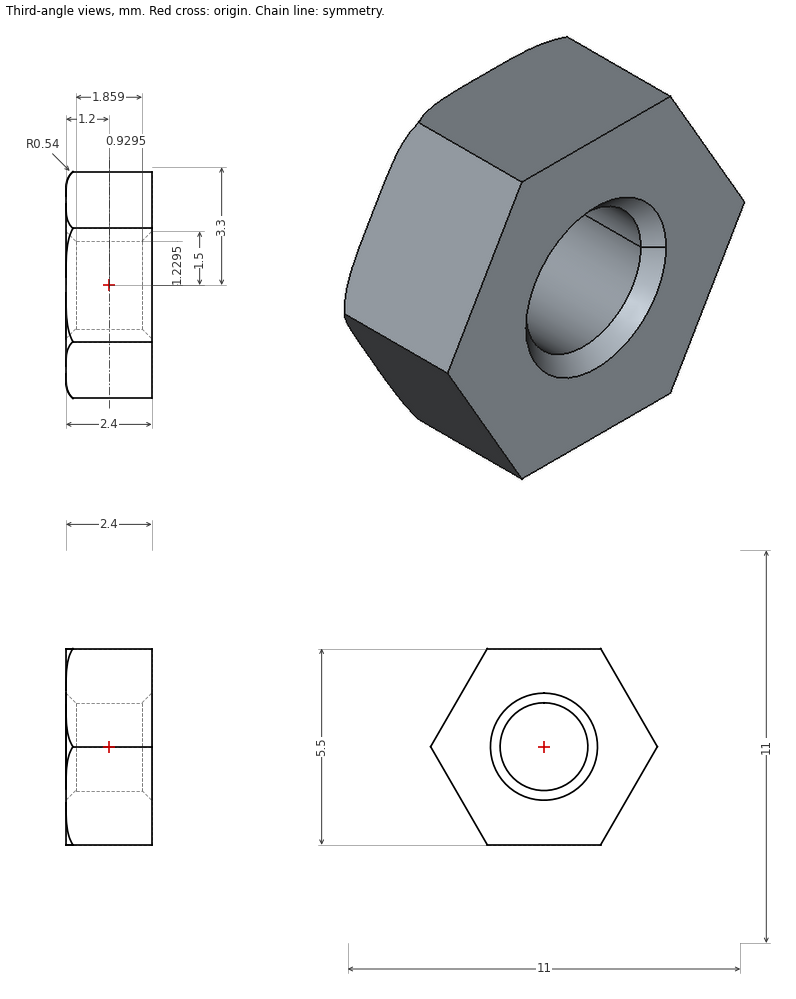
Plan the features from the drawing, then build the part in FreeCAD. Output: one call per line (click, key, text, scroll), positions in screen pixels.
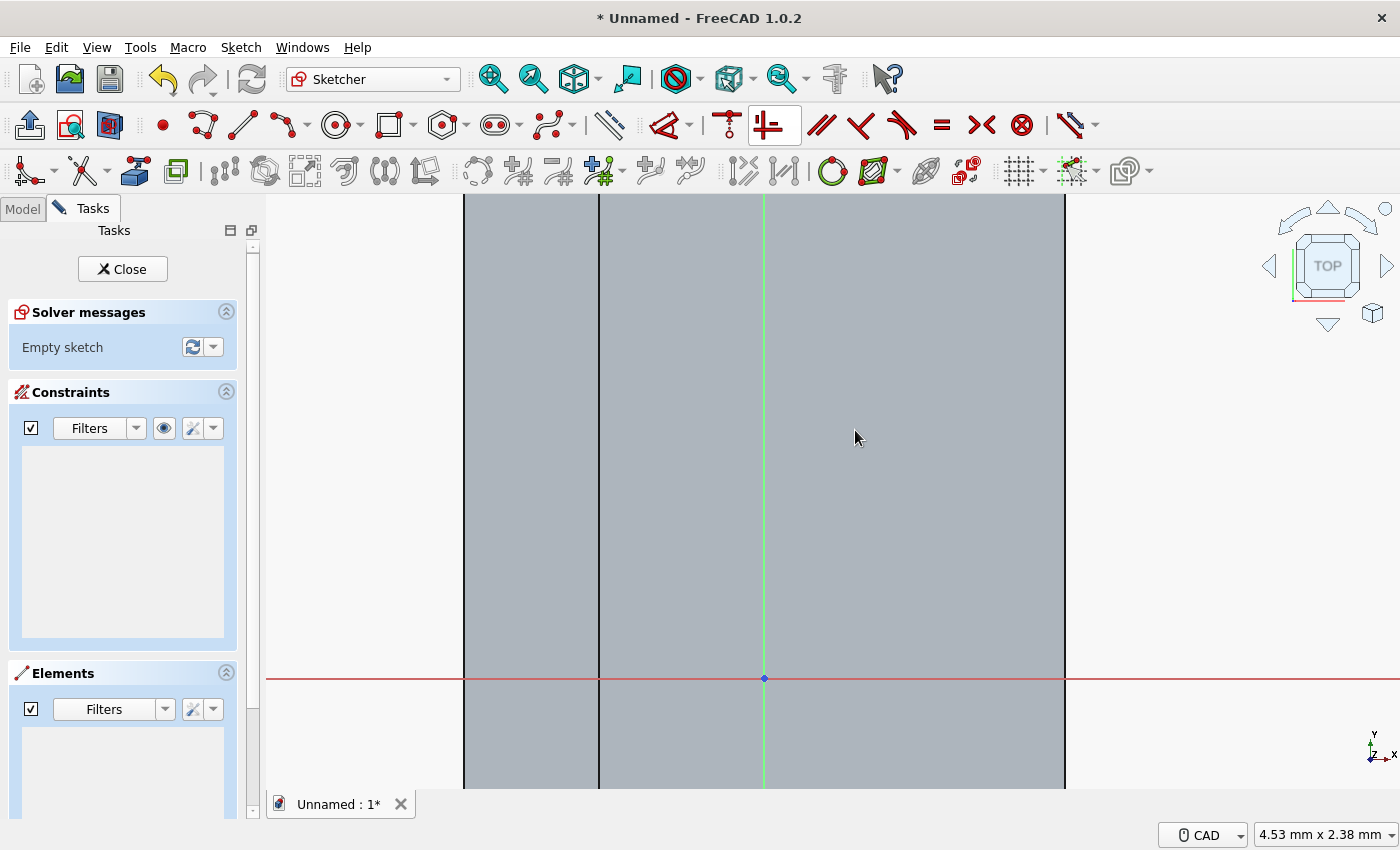
click(204, 126)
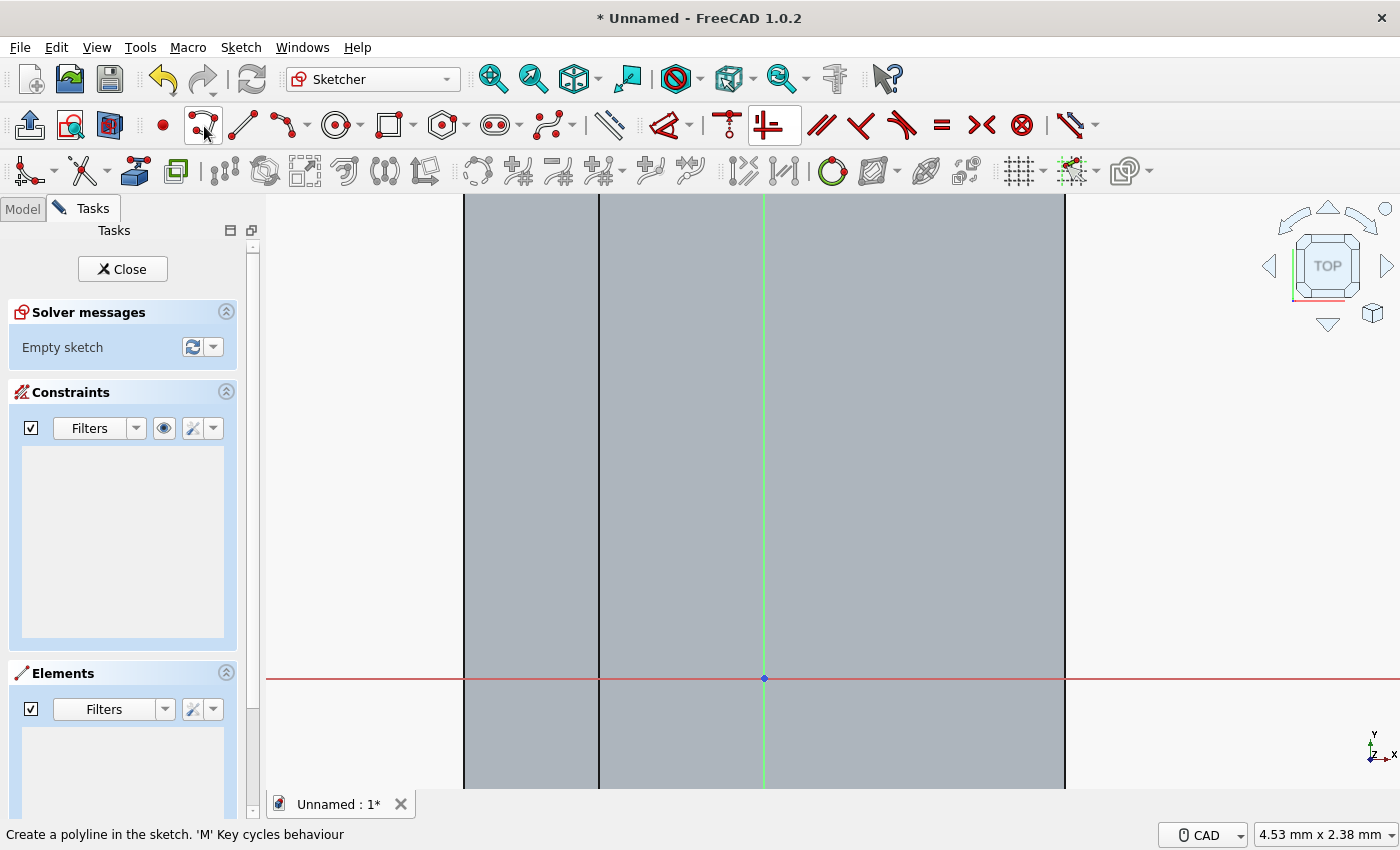
click(464, 679)
click(1065, 670)
click(1065, 303)
click(997, 371)
click(531, 371)
click(464, 303)
click(464, 679)
key(Escape)
key(Escape)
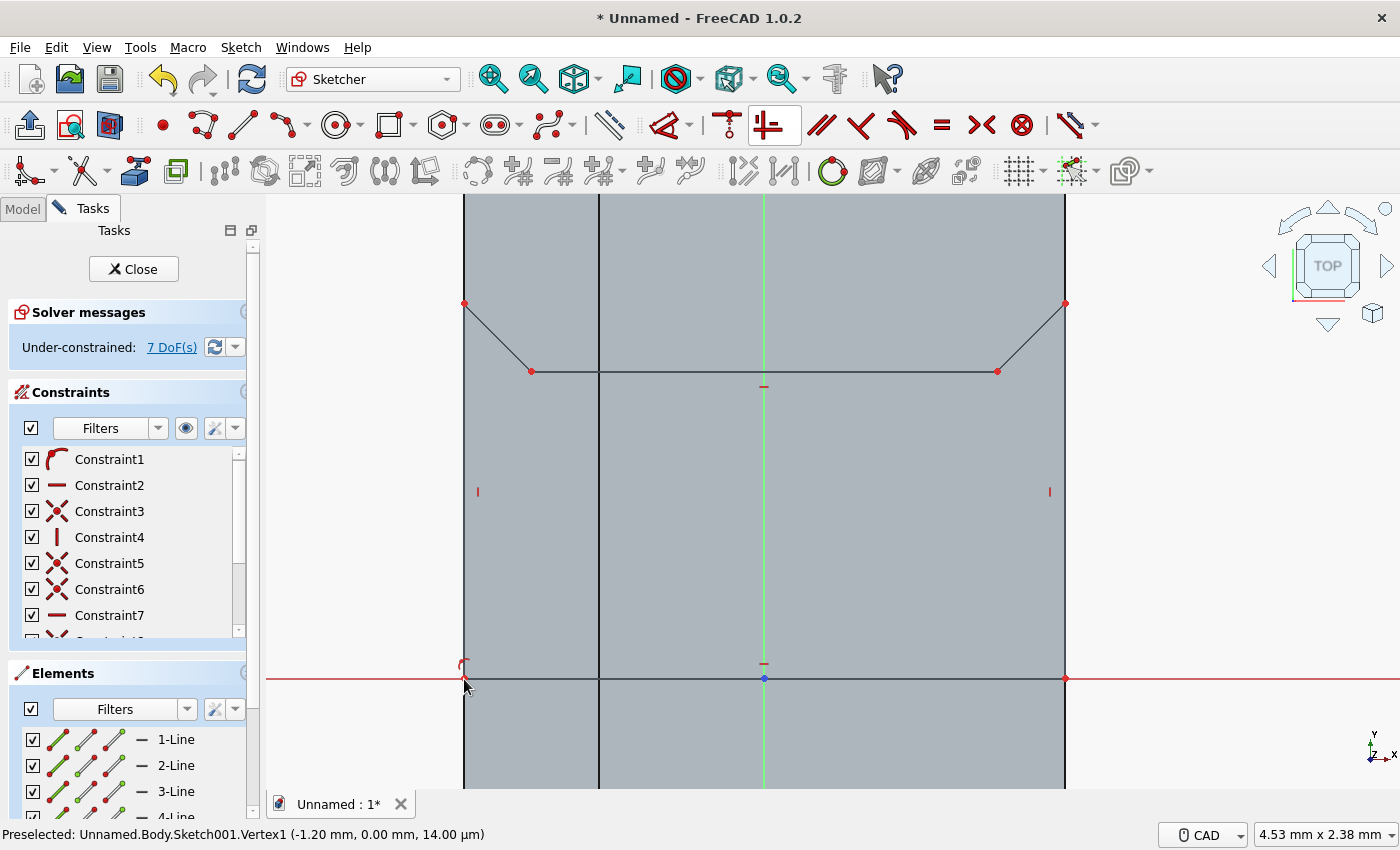
click(1065, 304)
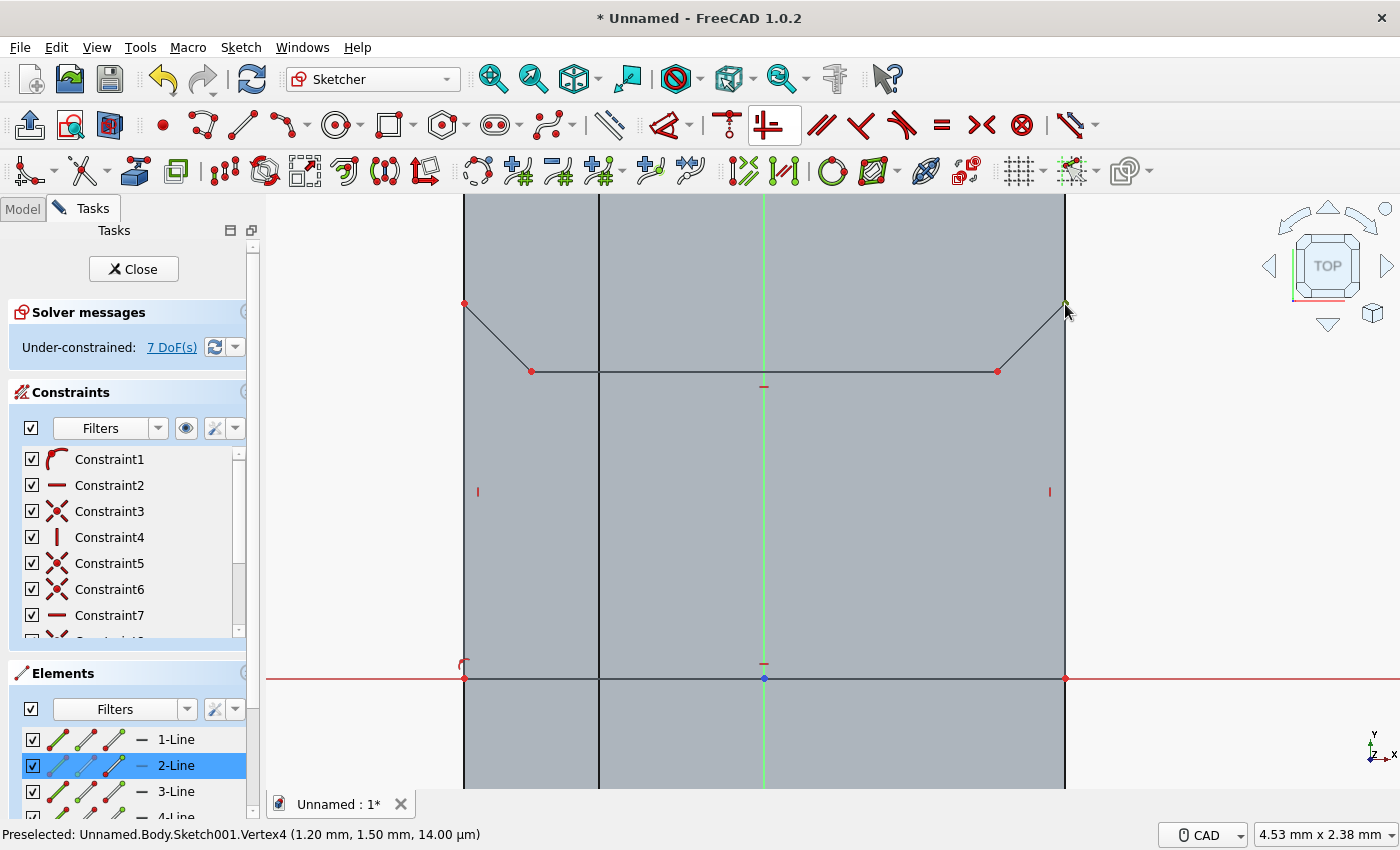
click(464, 304)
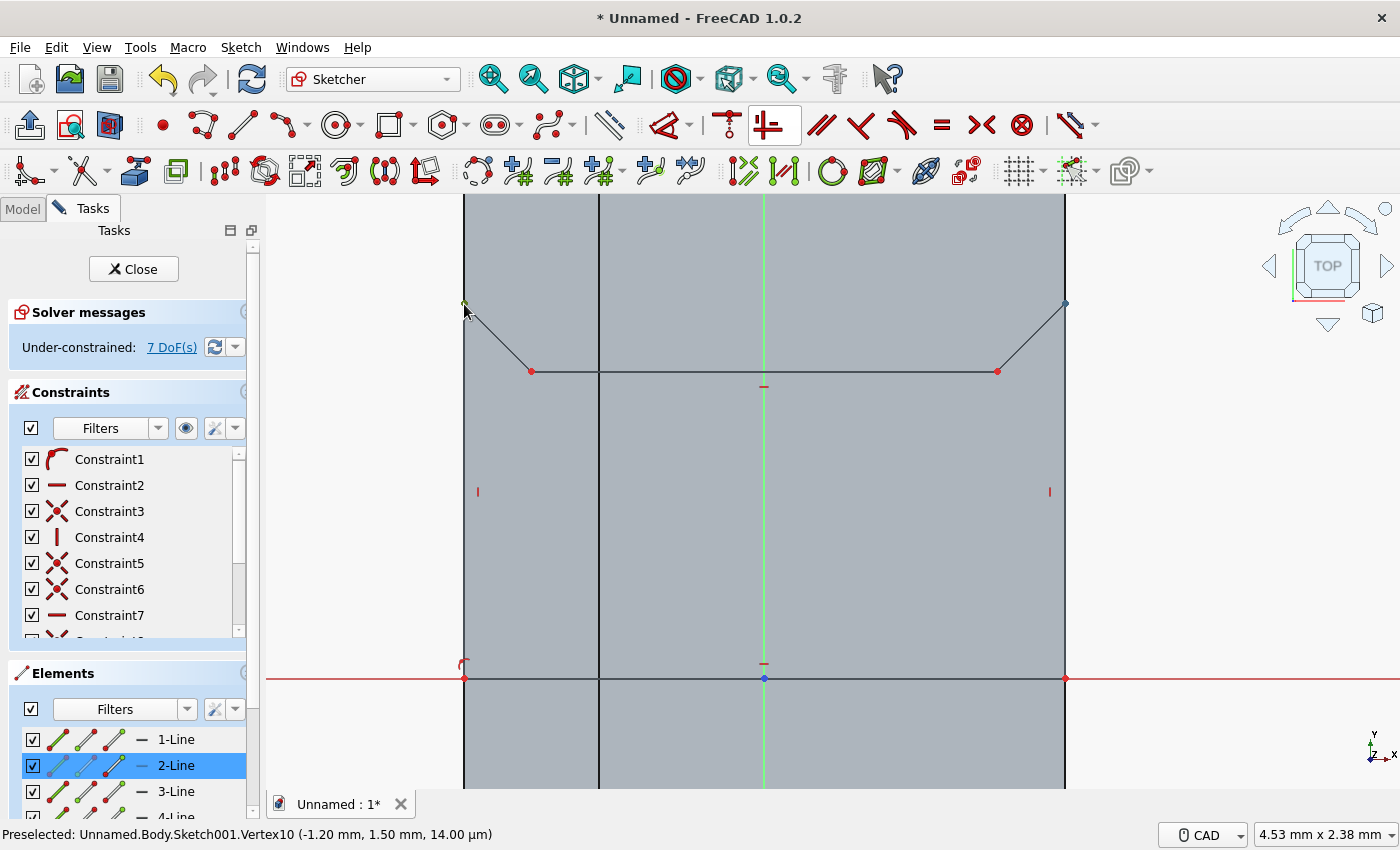
click(764, 722)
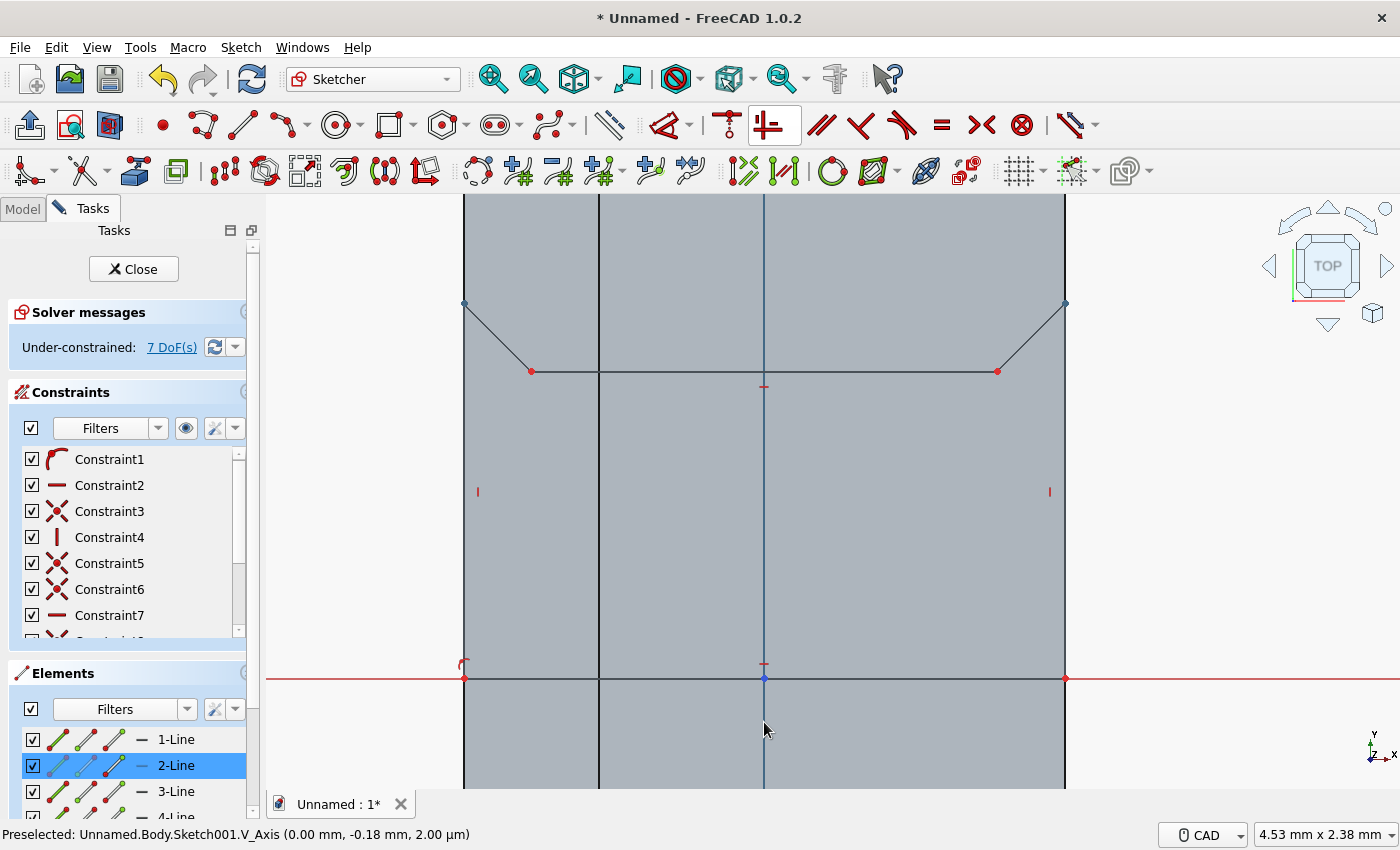
click(982, 126)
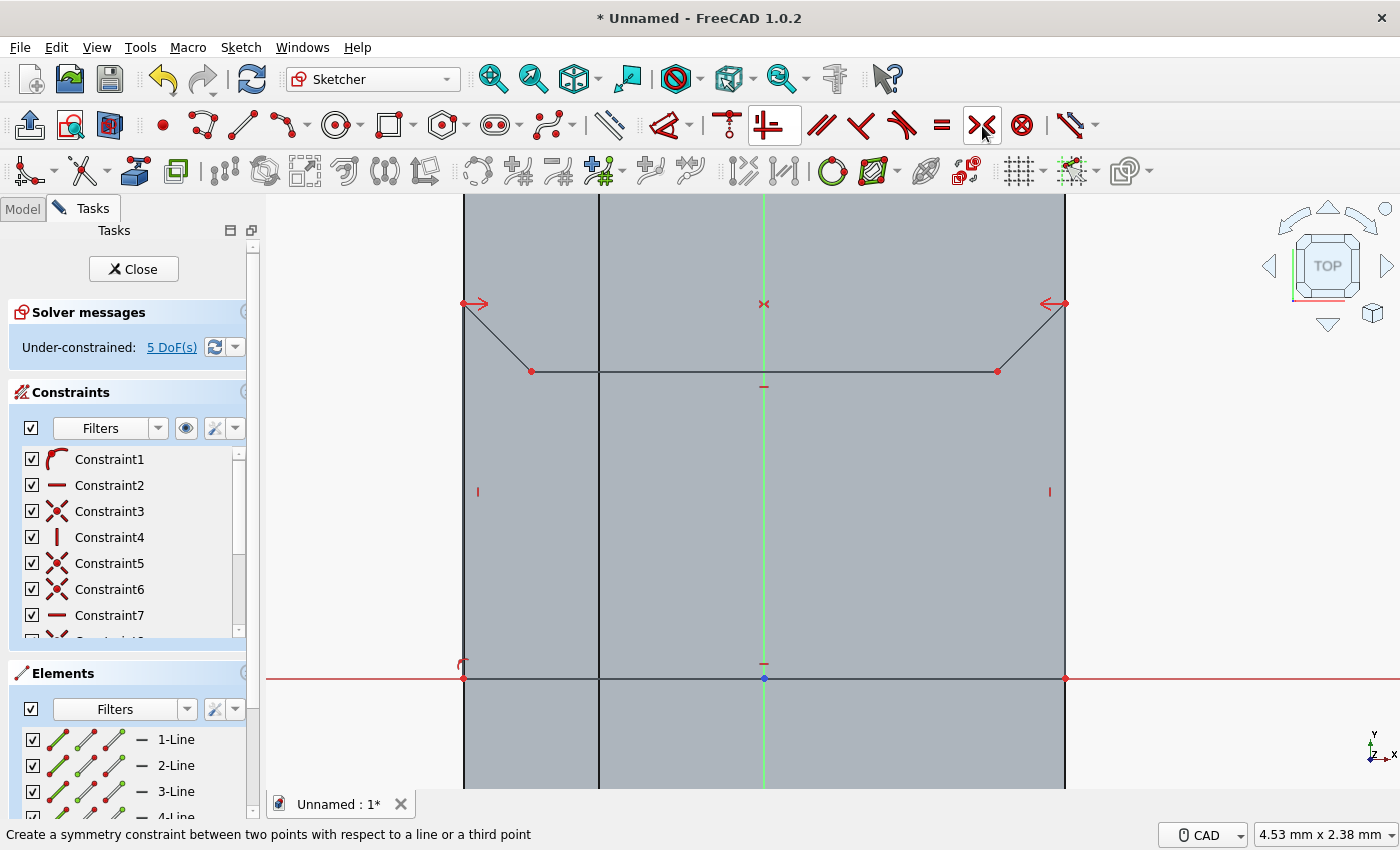
click(664, 126)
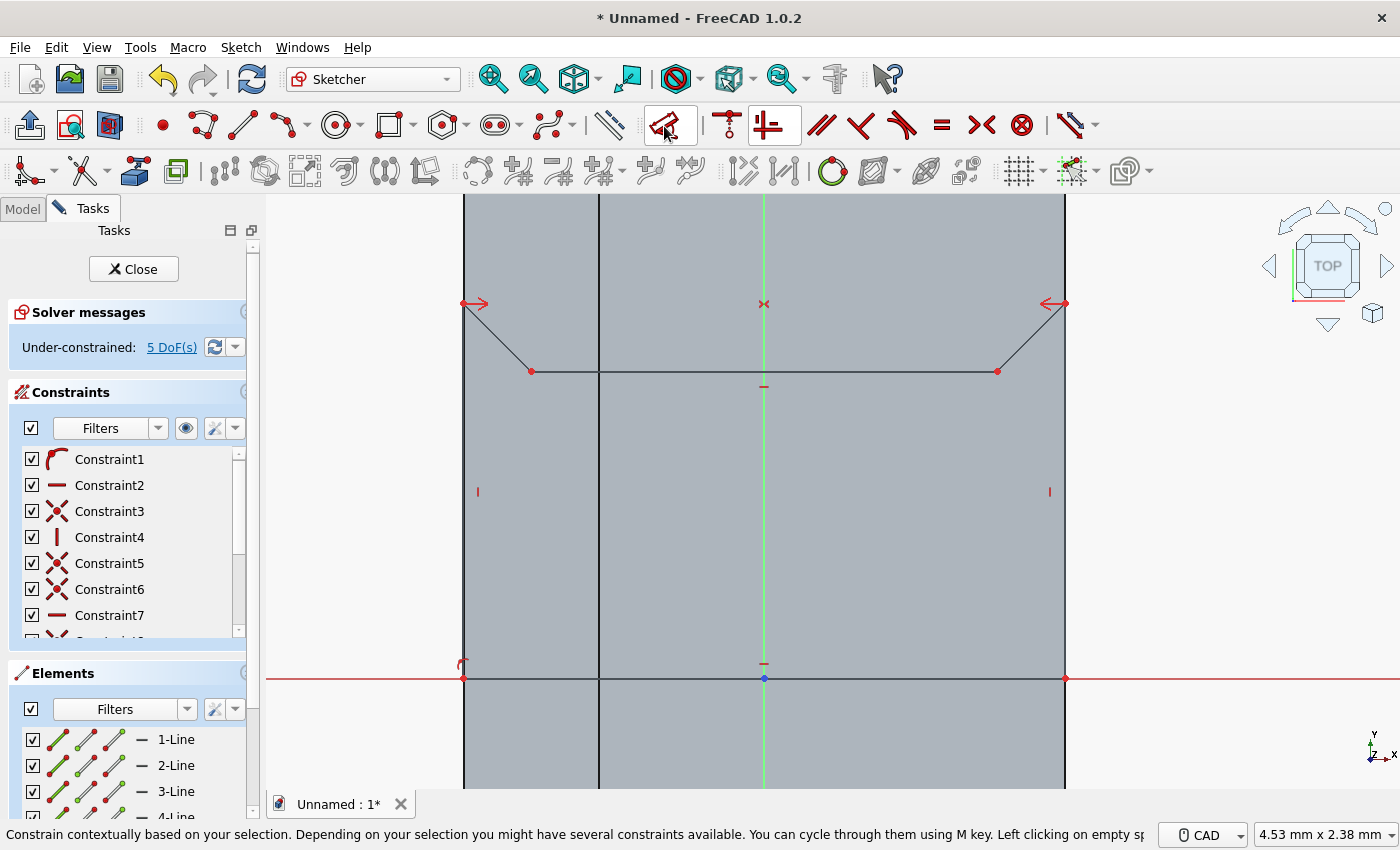
click(644, 679)
click(626, 713)